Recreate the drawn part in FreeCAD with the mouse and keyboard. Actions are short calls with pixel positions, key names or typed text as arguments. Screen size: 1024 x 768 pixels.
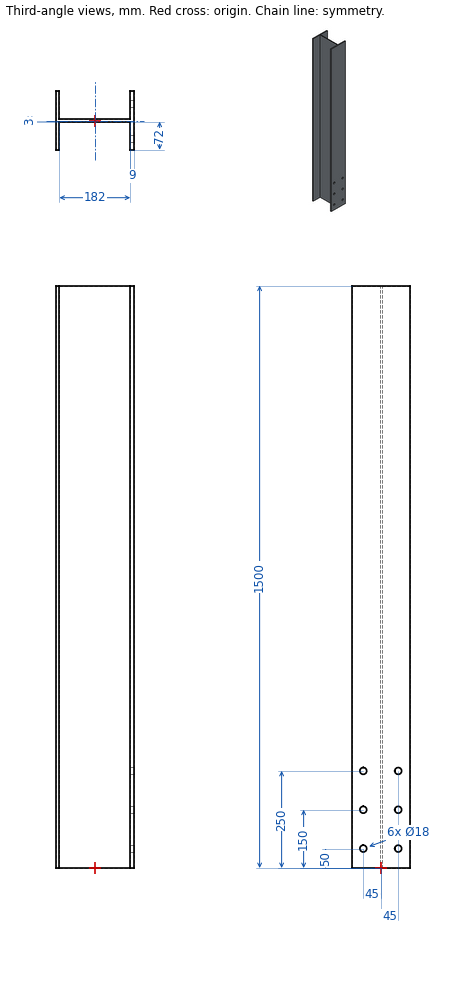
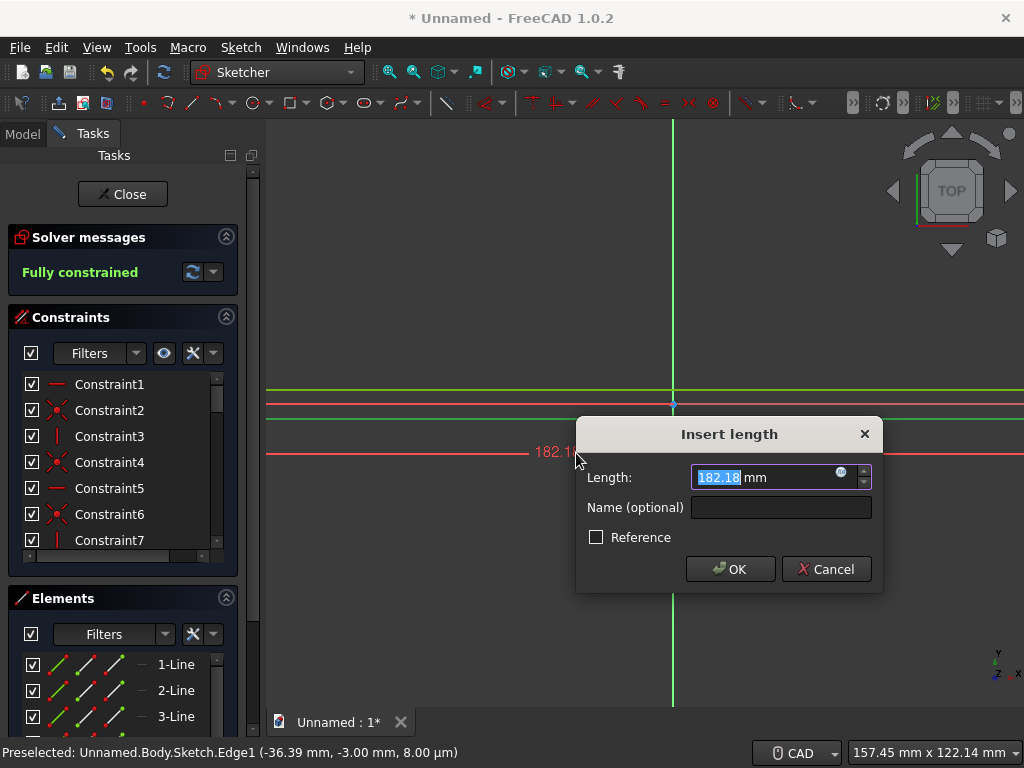
text(182)
key(Return)
key(Escape)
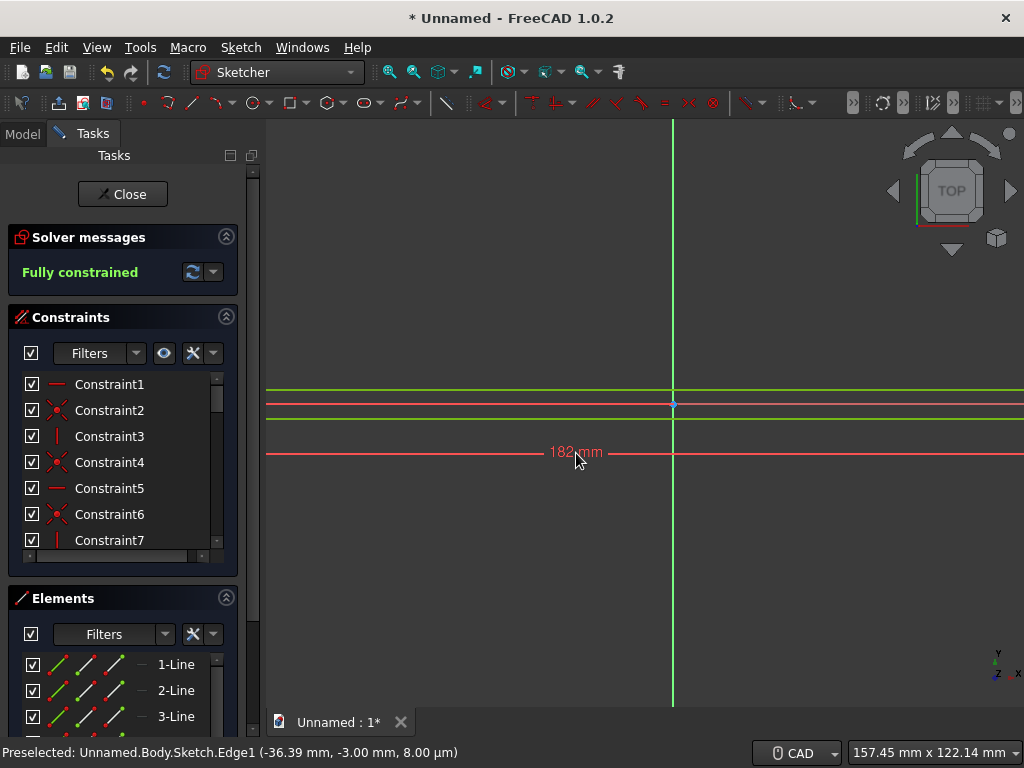
click(123, 194)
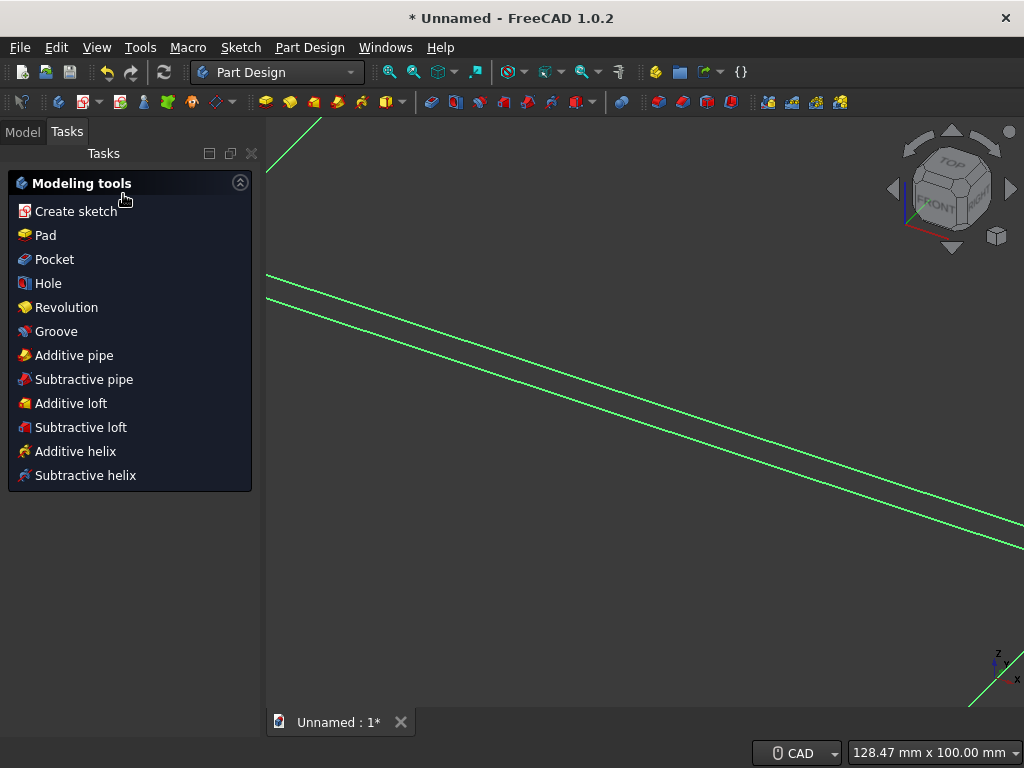
click(266, 102)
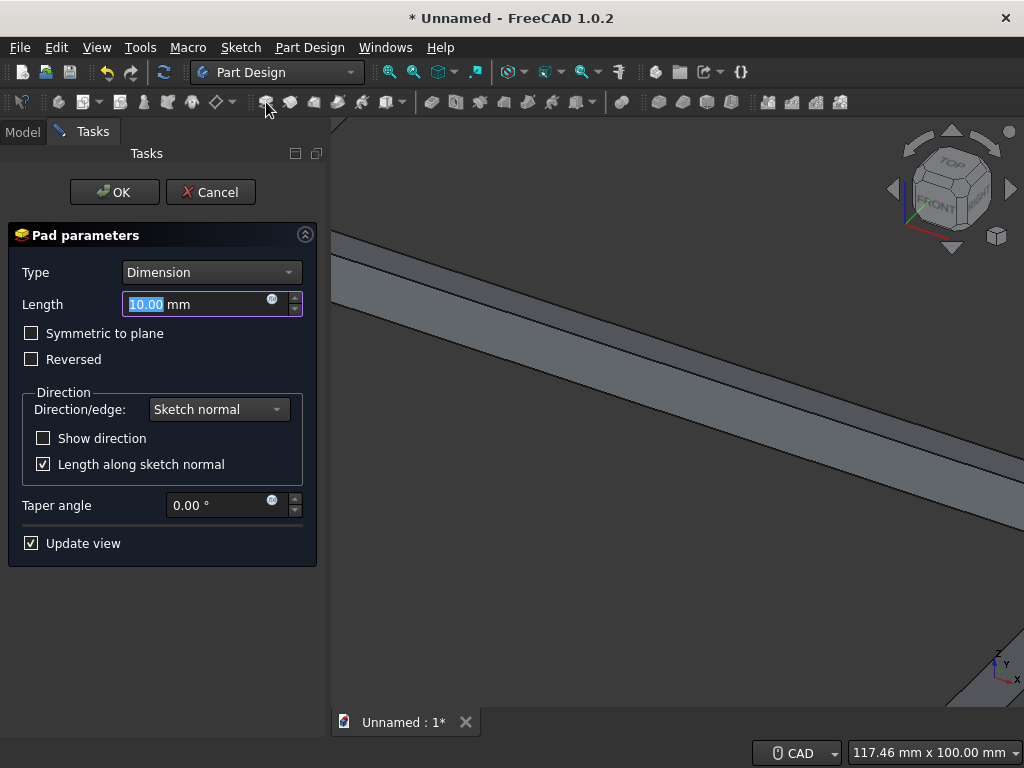
text(1500)
key(Tab)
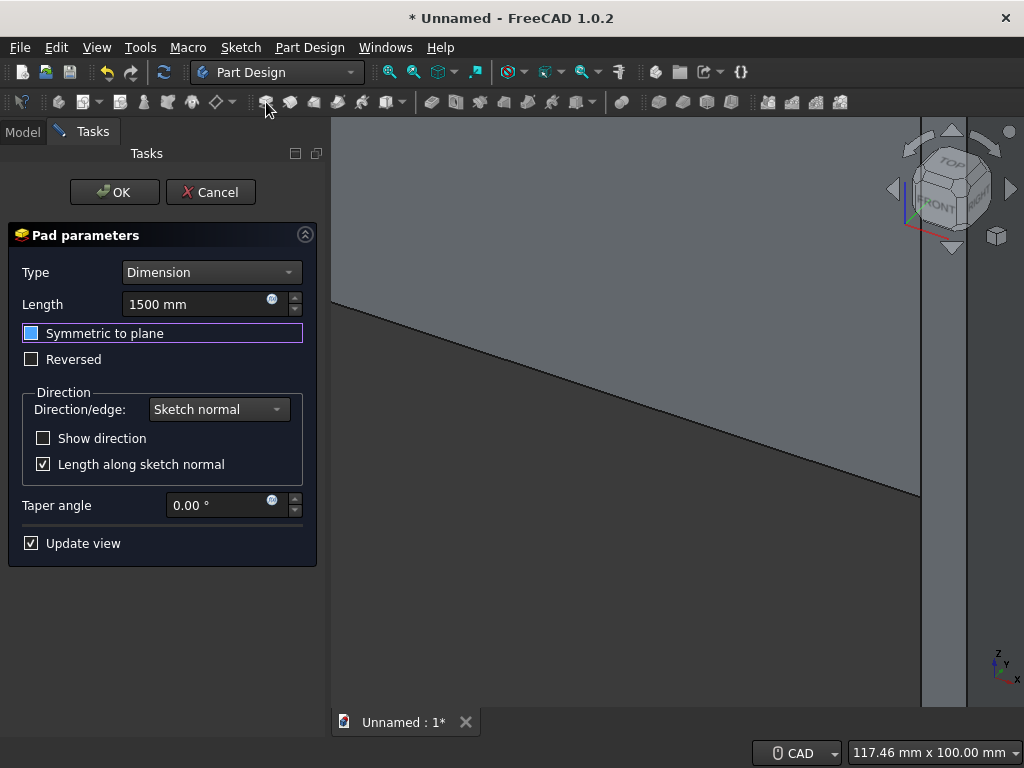
click(115, 192)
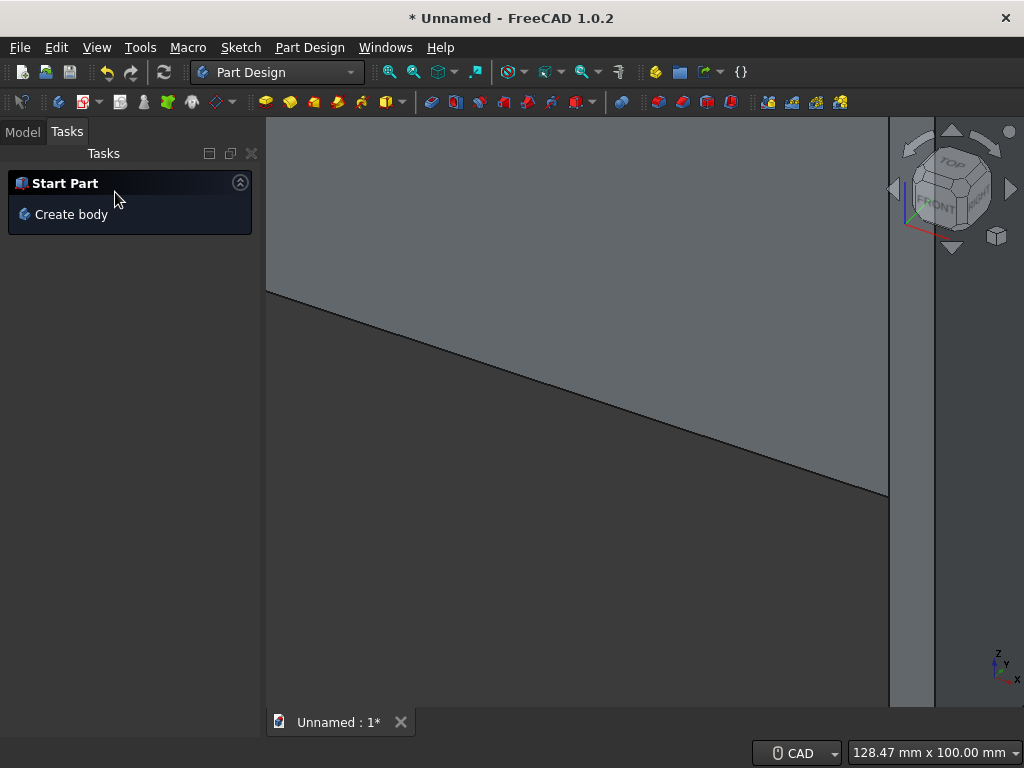
click(390, 72)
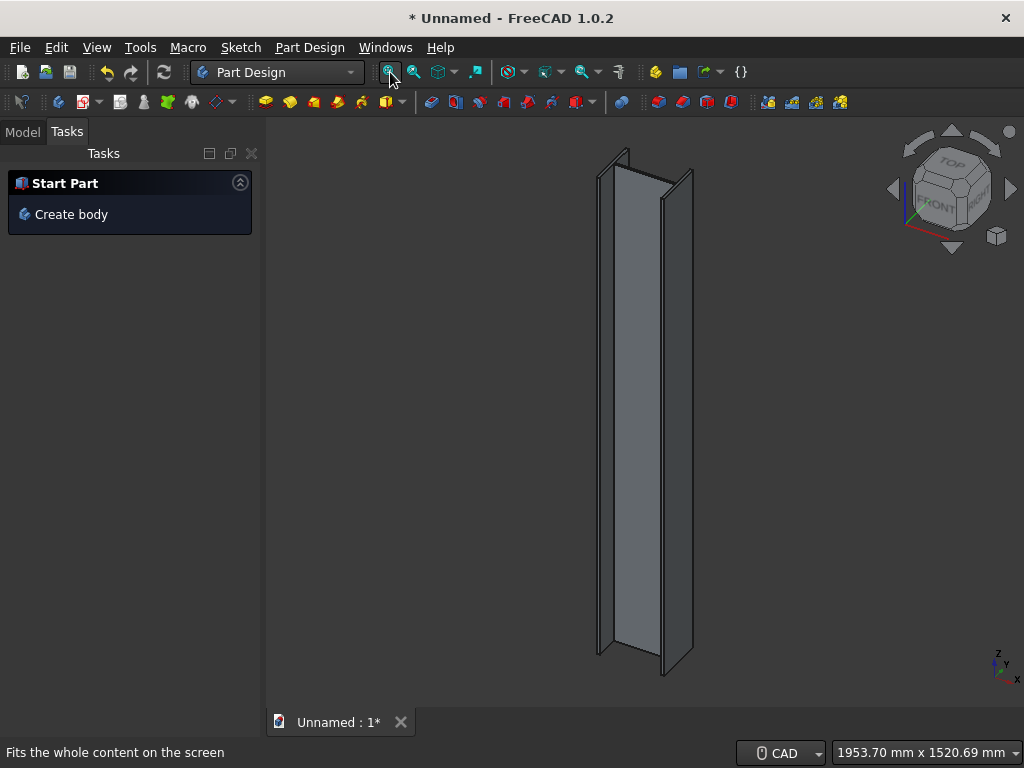
click(23, 131)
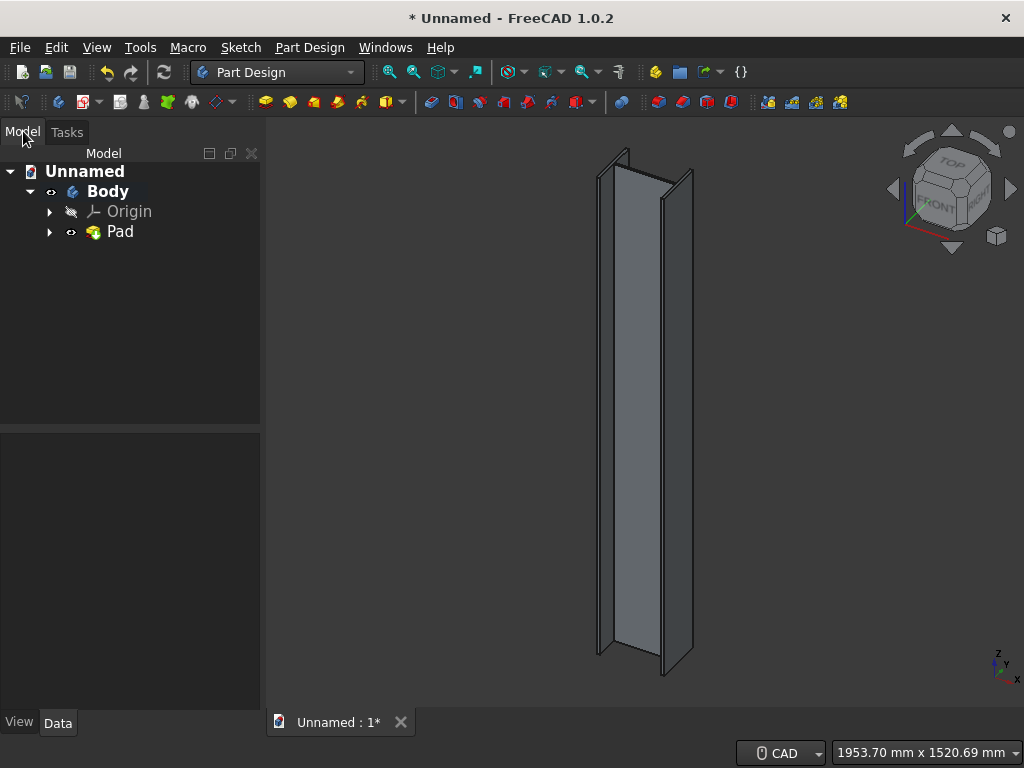
click(50, 212)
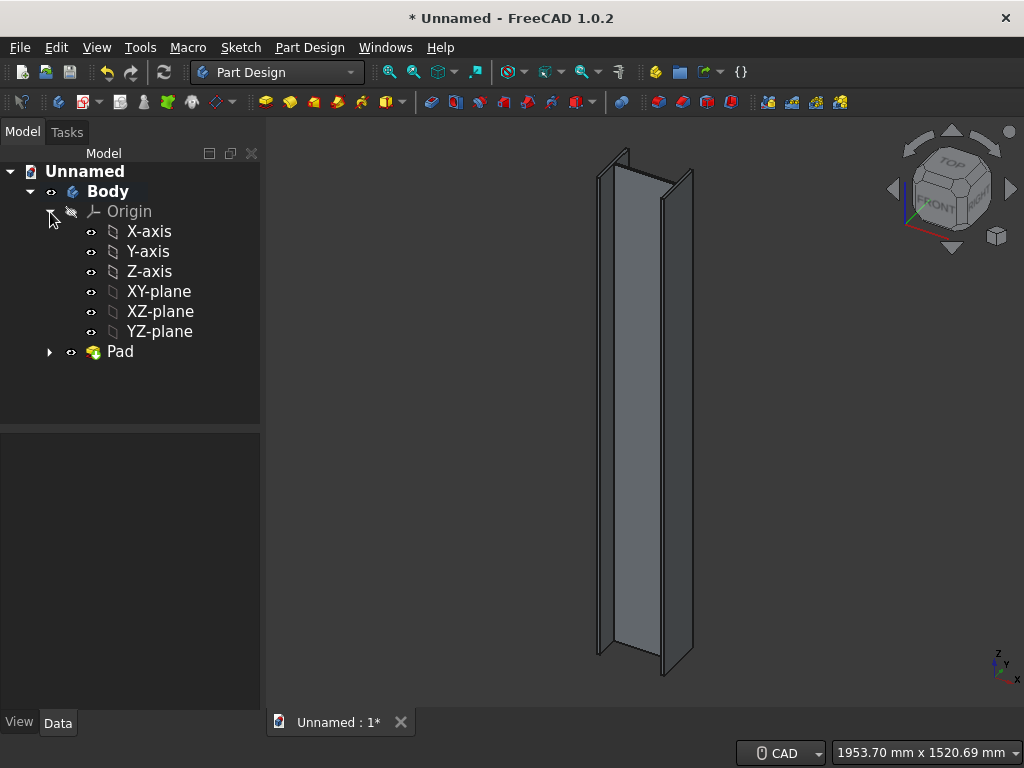
click(136, 332)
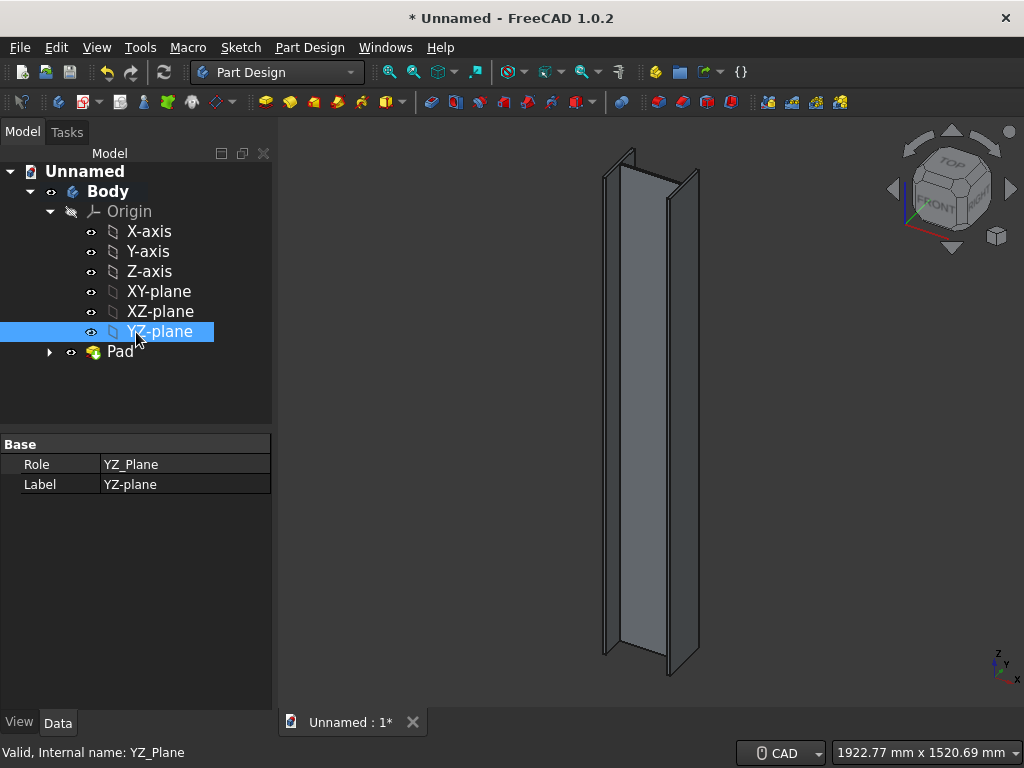
click(216, 102)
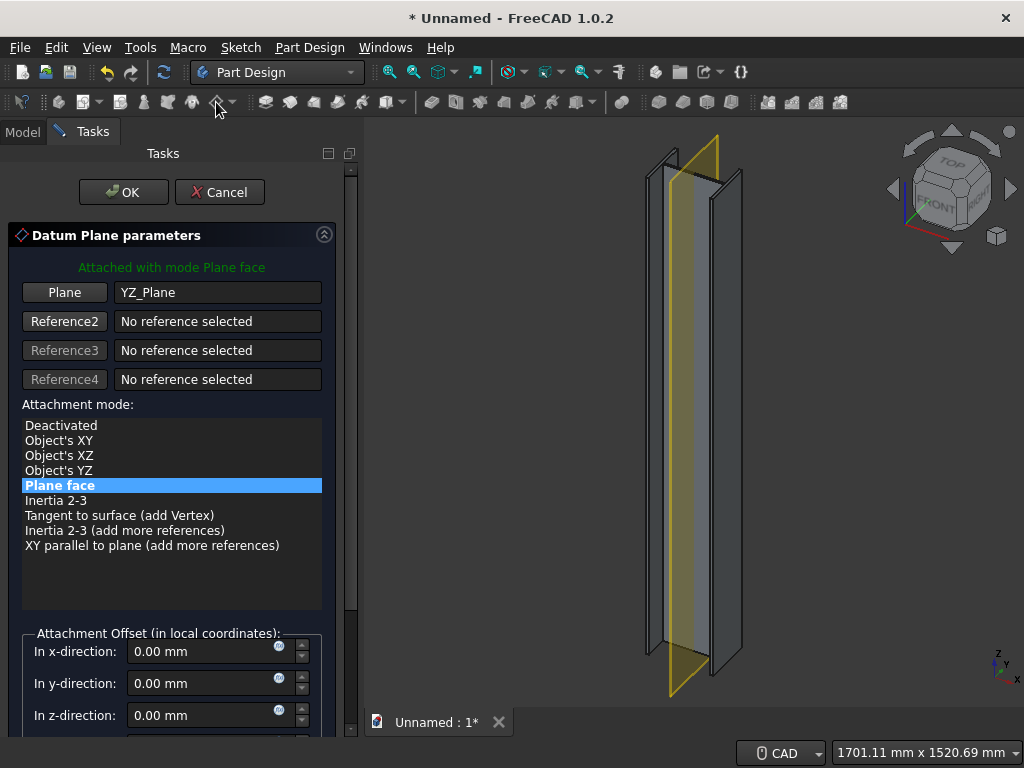
triple_click(210, 715)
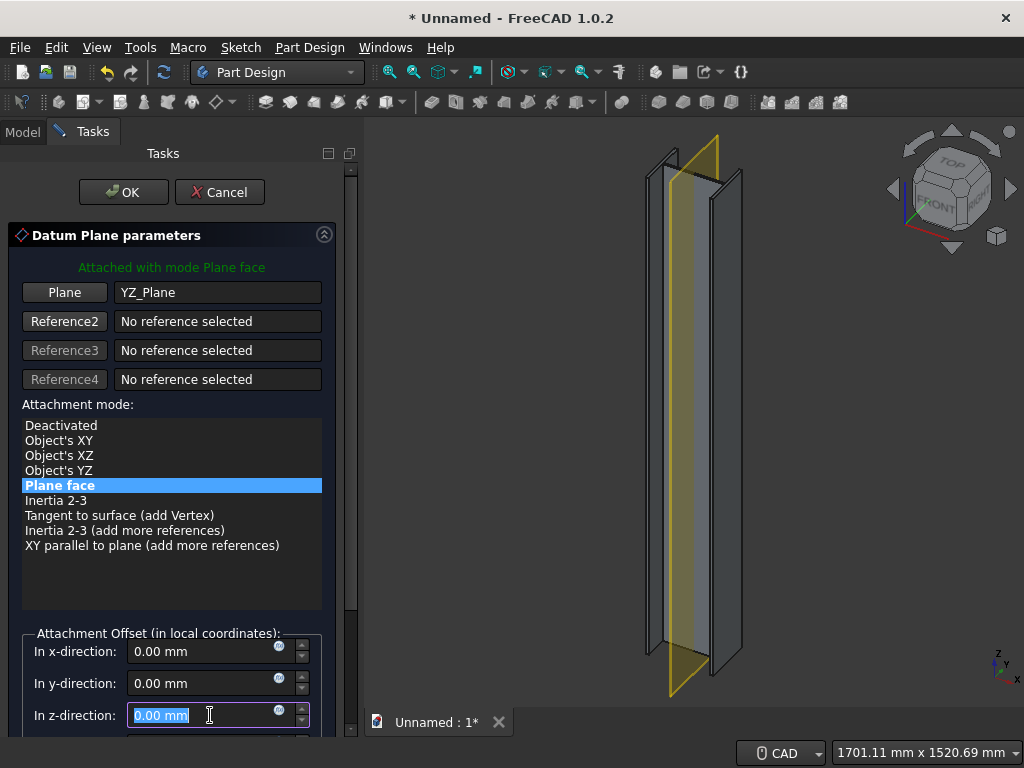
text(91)
key(Tab)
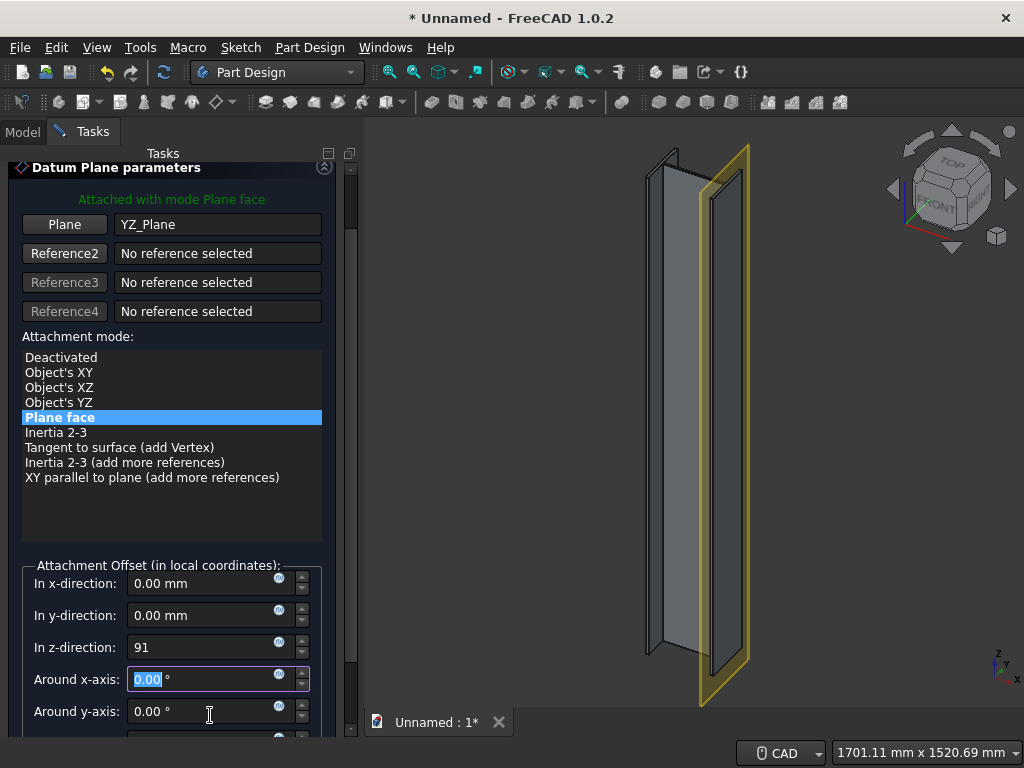
scroll(351, 450, up, 2)